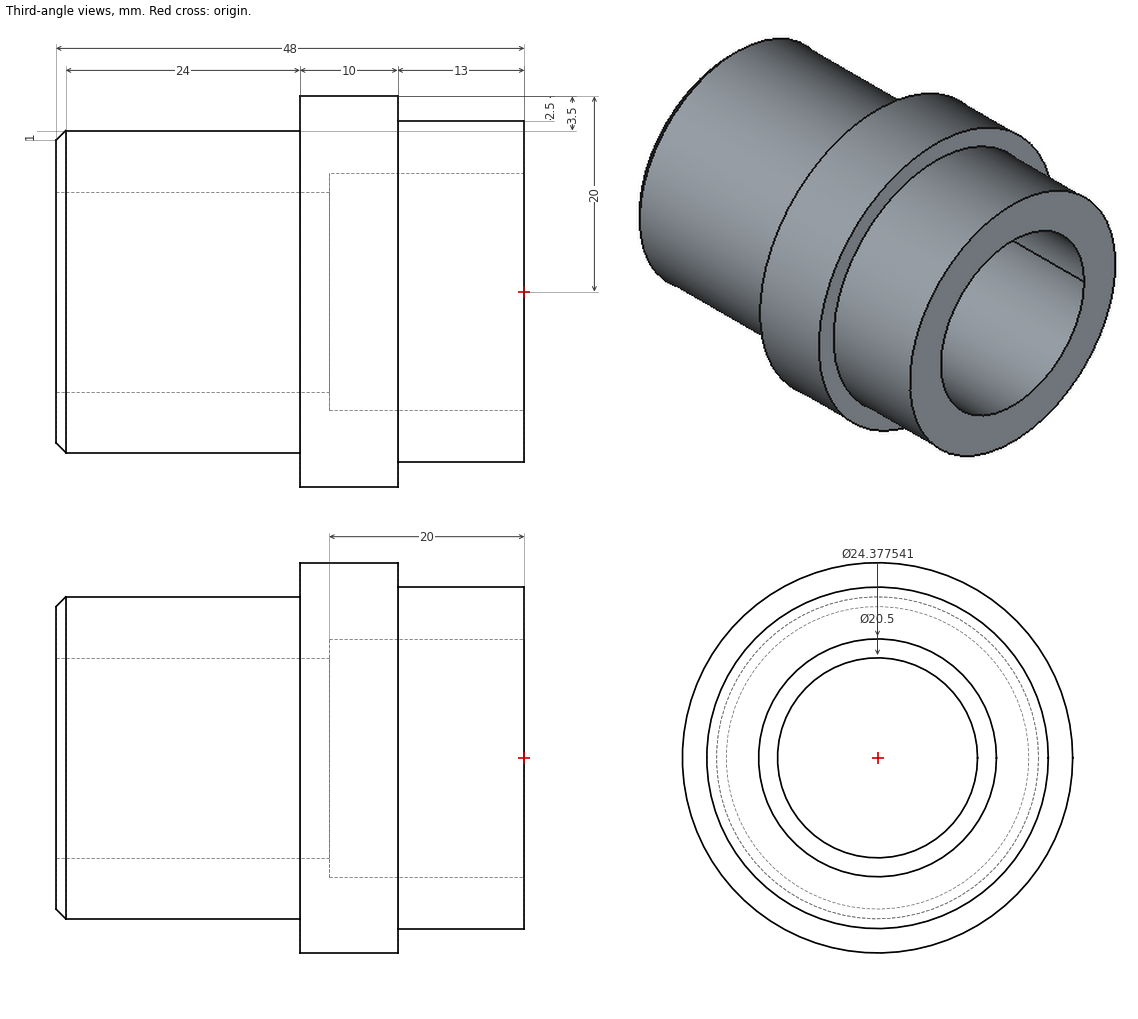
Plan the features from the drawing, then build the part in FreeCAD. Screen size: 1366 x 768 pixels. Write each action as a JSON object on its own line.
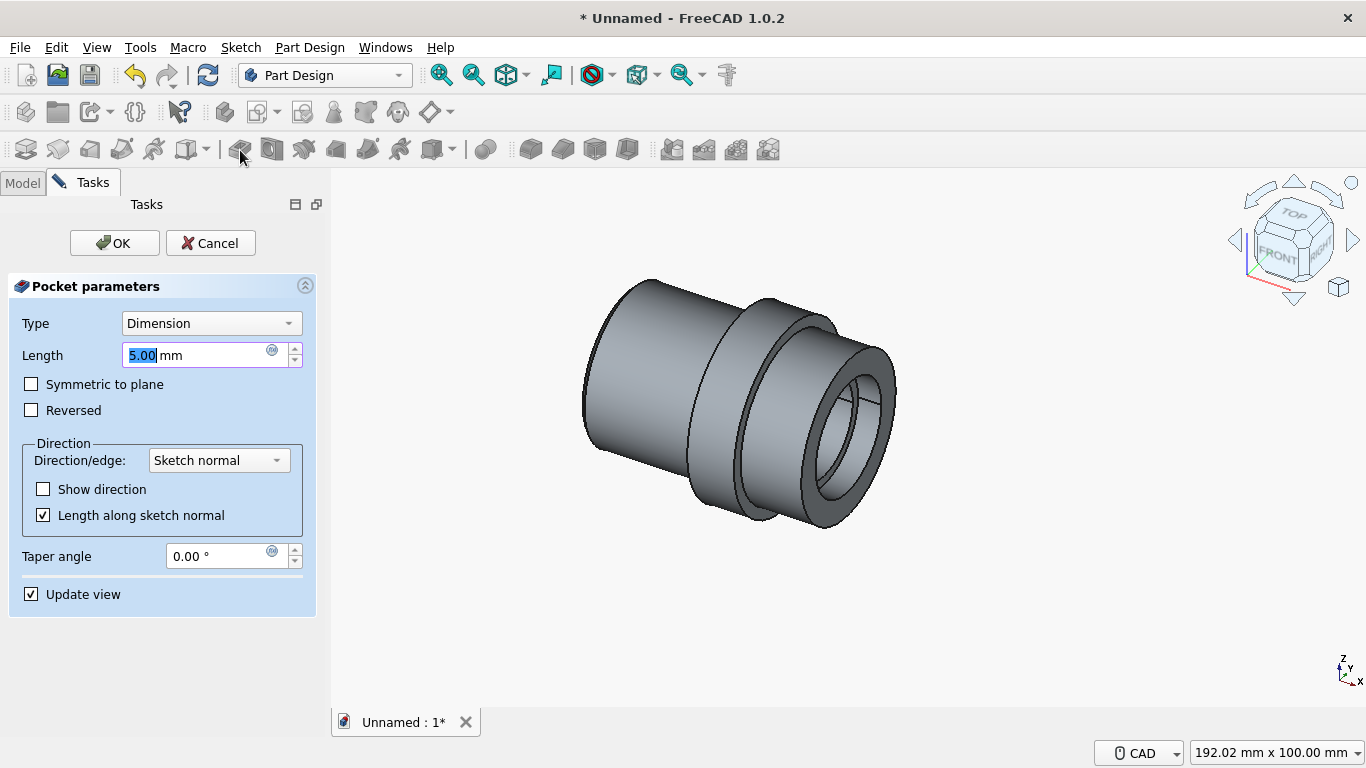
{"action": "type", "text": "20"}
{"action": "key", "text": "Tab"}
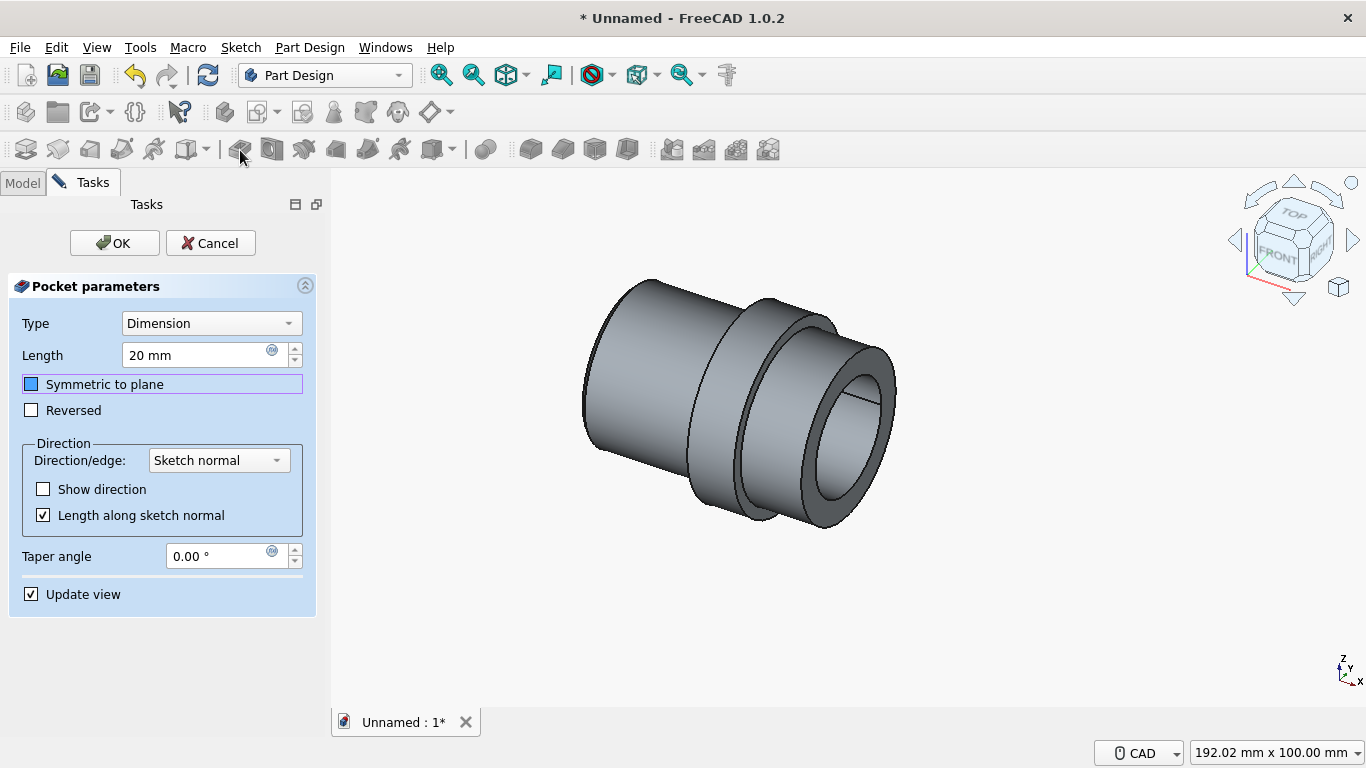
{"action": "left_click", "coordinate": [115, 243]}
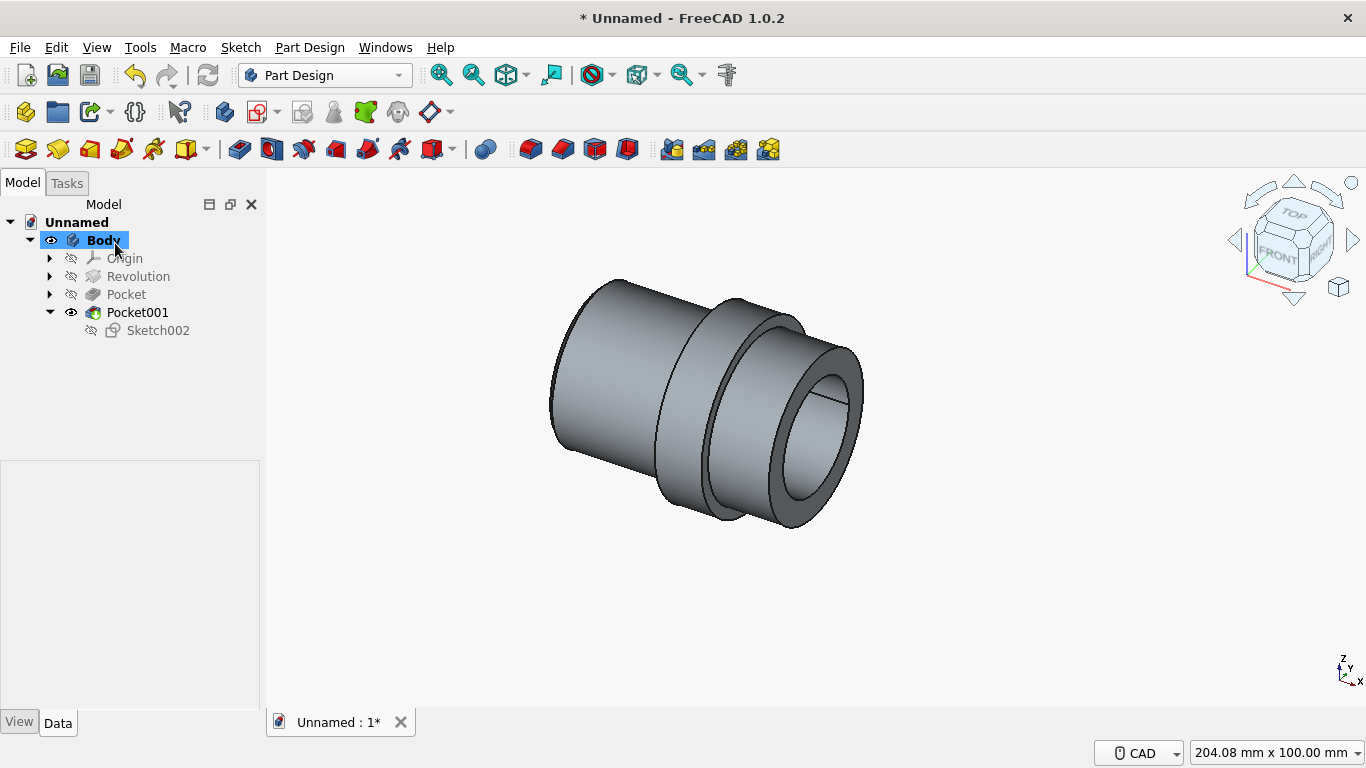
{"action": "key", "text": "0"}